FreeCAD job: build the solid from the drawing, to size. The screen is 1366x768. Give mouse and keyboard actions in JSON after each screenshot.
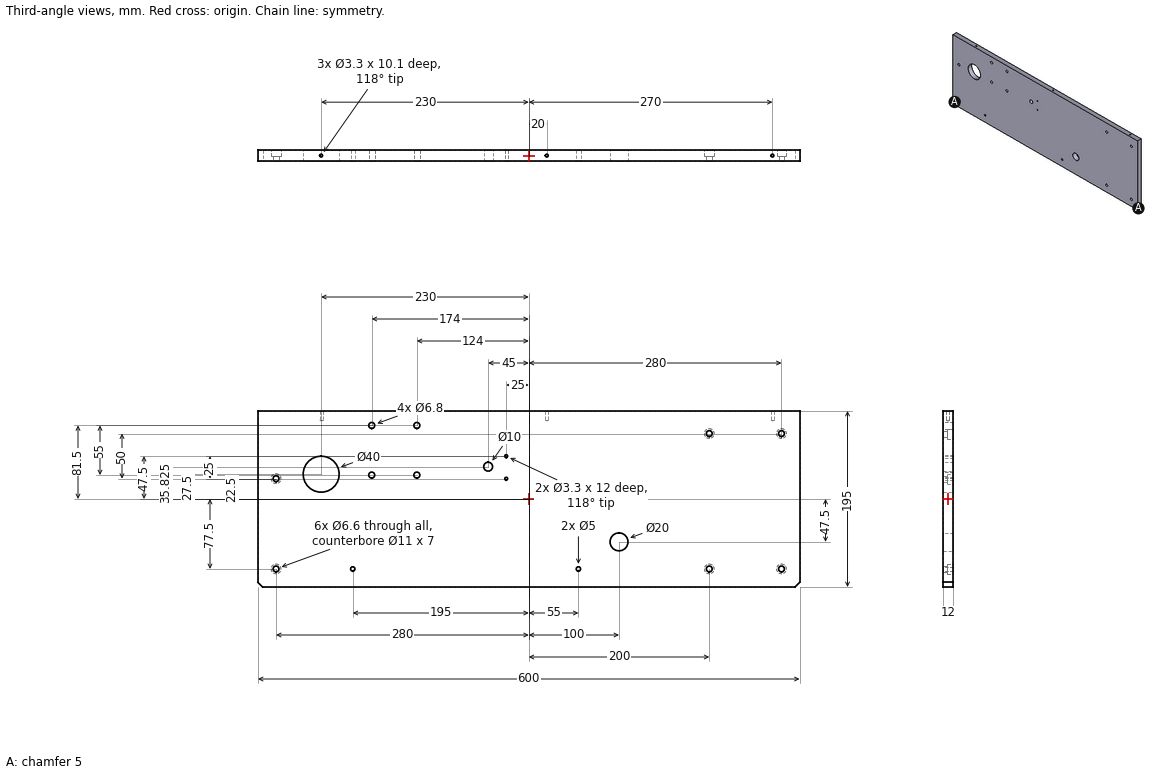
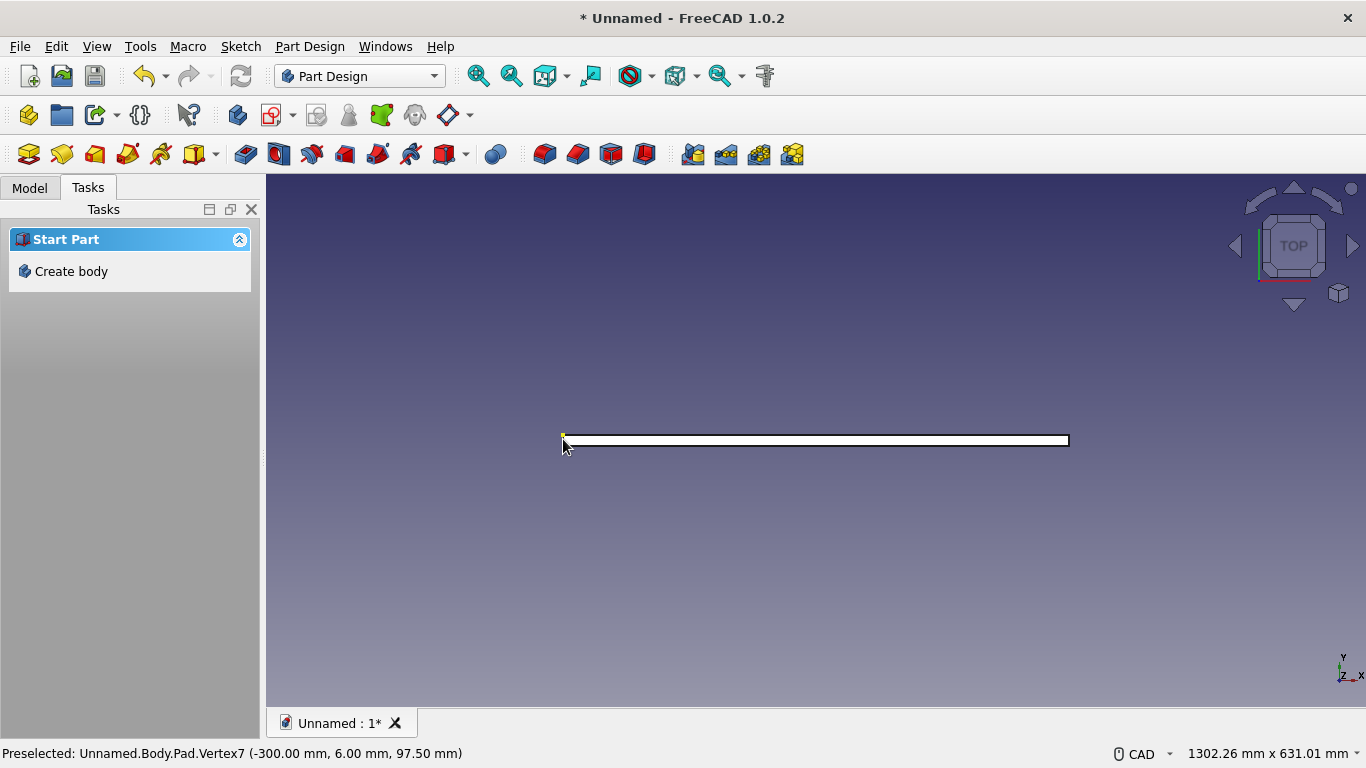
{"action": "key", "text": "1"}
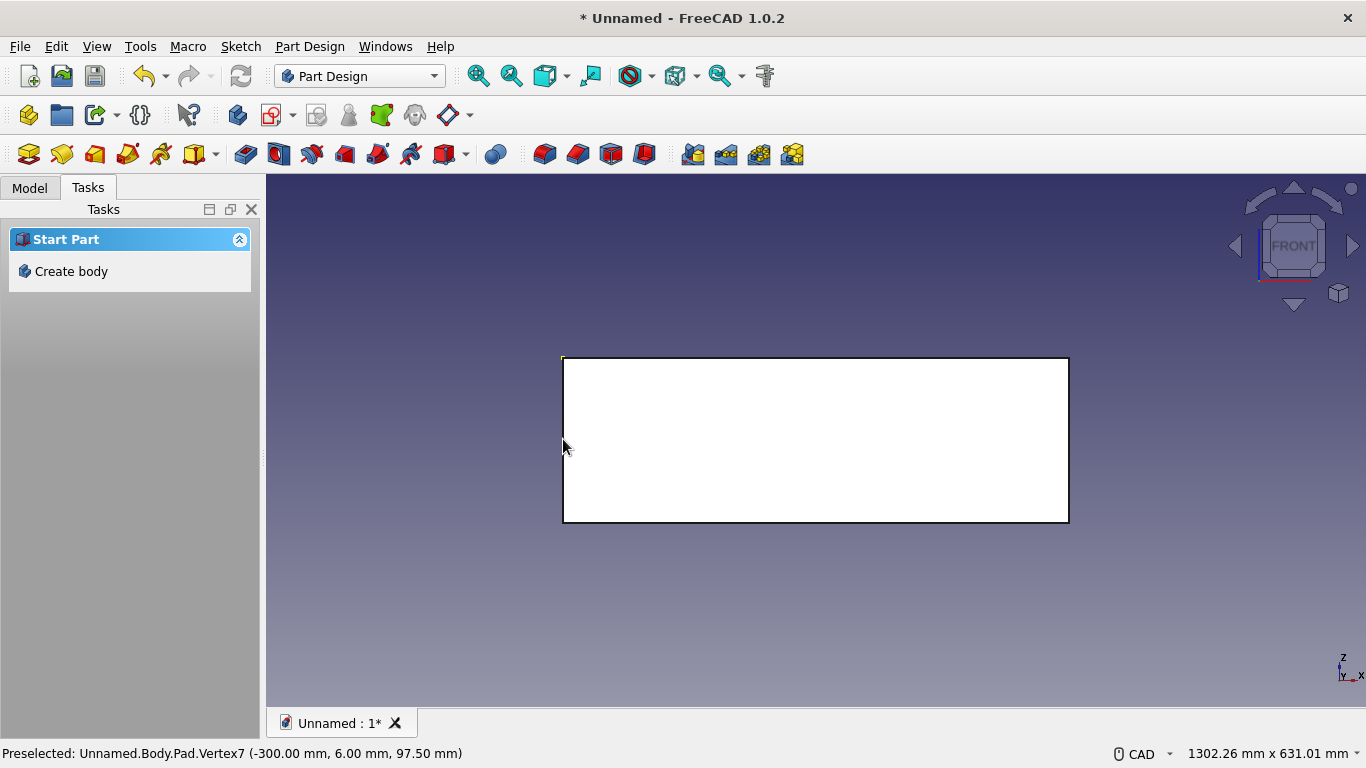
{"action": "scroll", "coordinate": [563, 522], "scroll_direction": "up", "scroll_amount": 7}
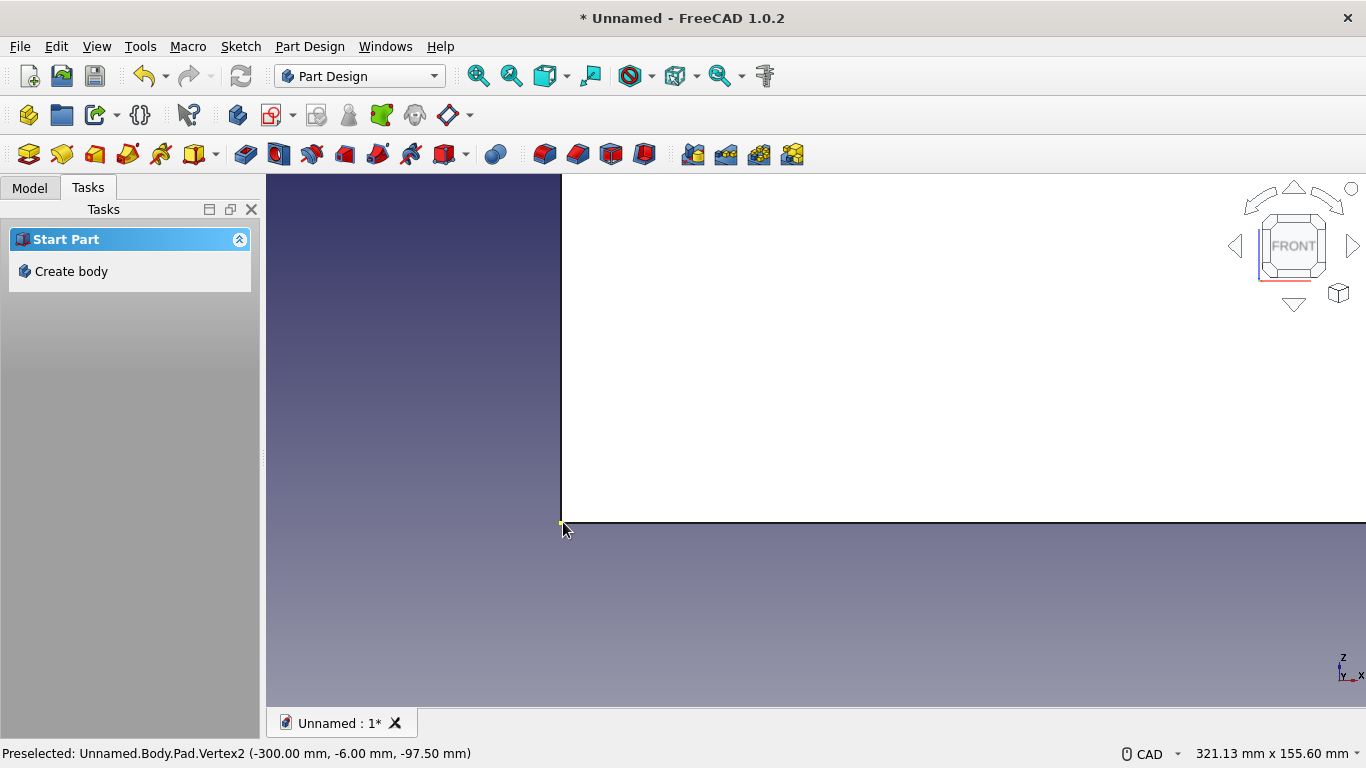
{"action": "key", "text": "v f"}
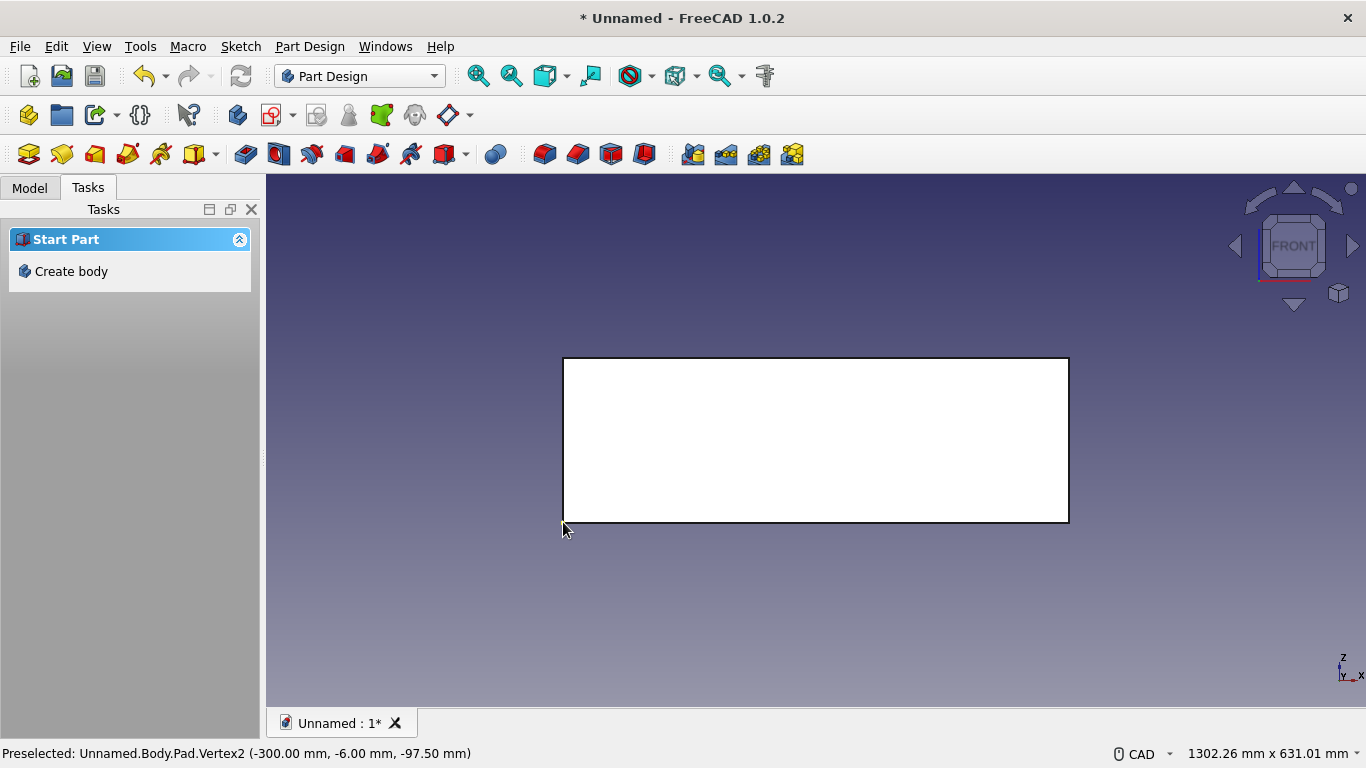
{"action": "key", "text": "3"}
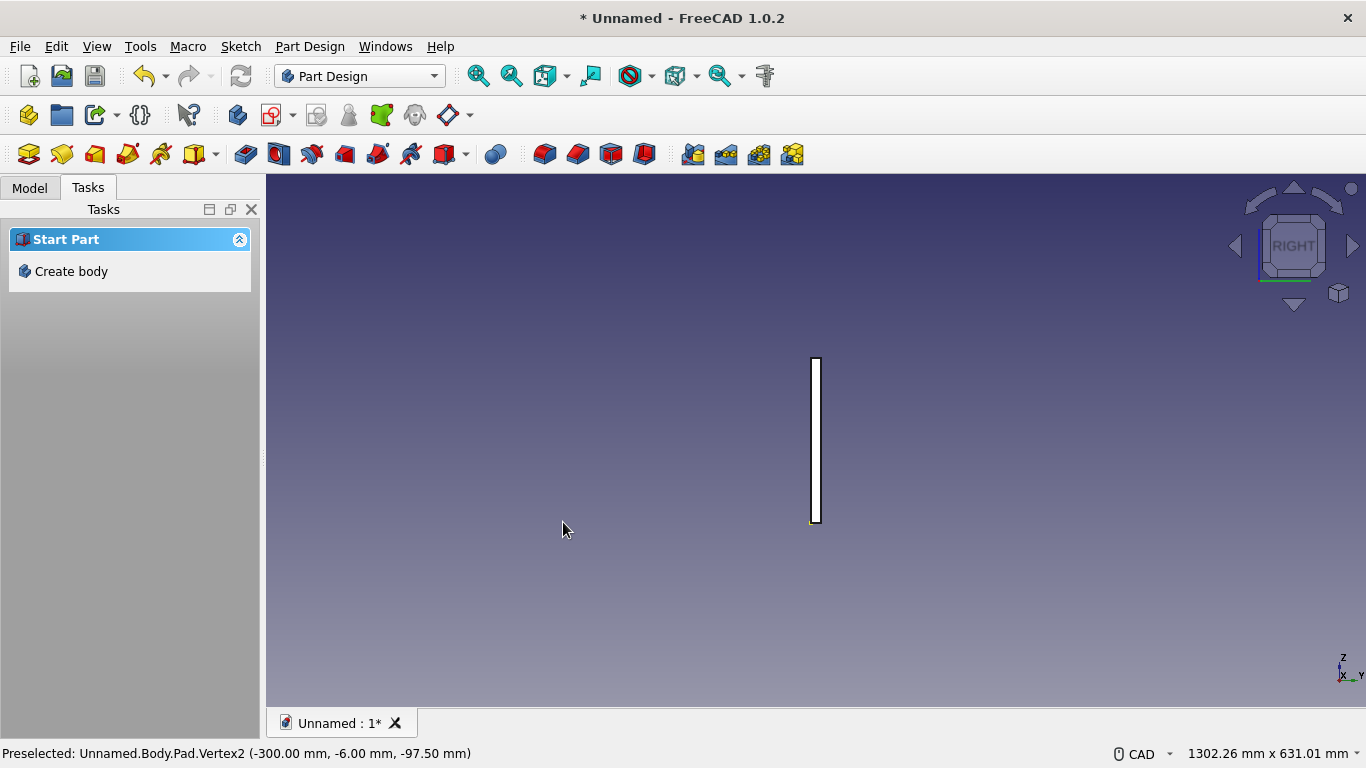
{"action": "key", "text": "v f"}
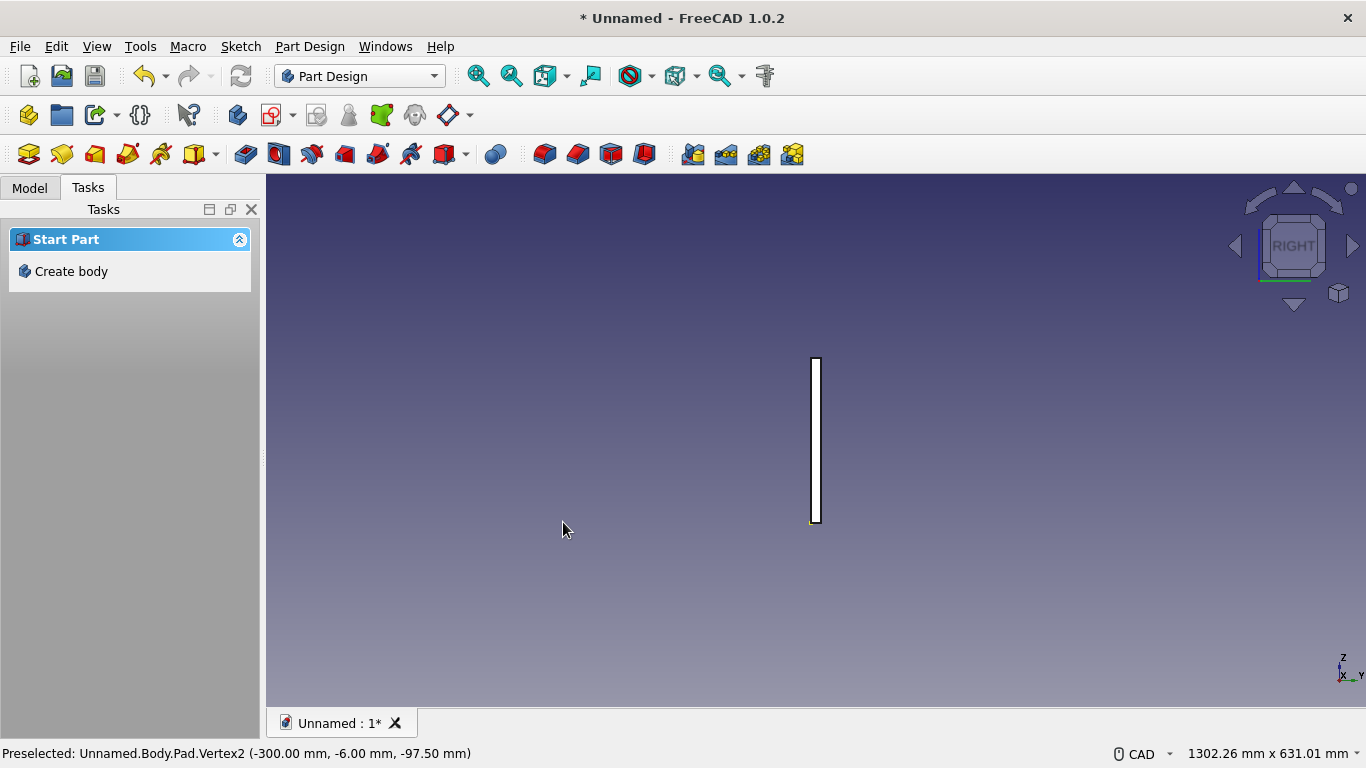
{"action": "scroll", "coordinate": [816, 522], "scroll_direction": "up", "scroll_amount": 7}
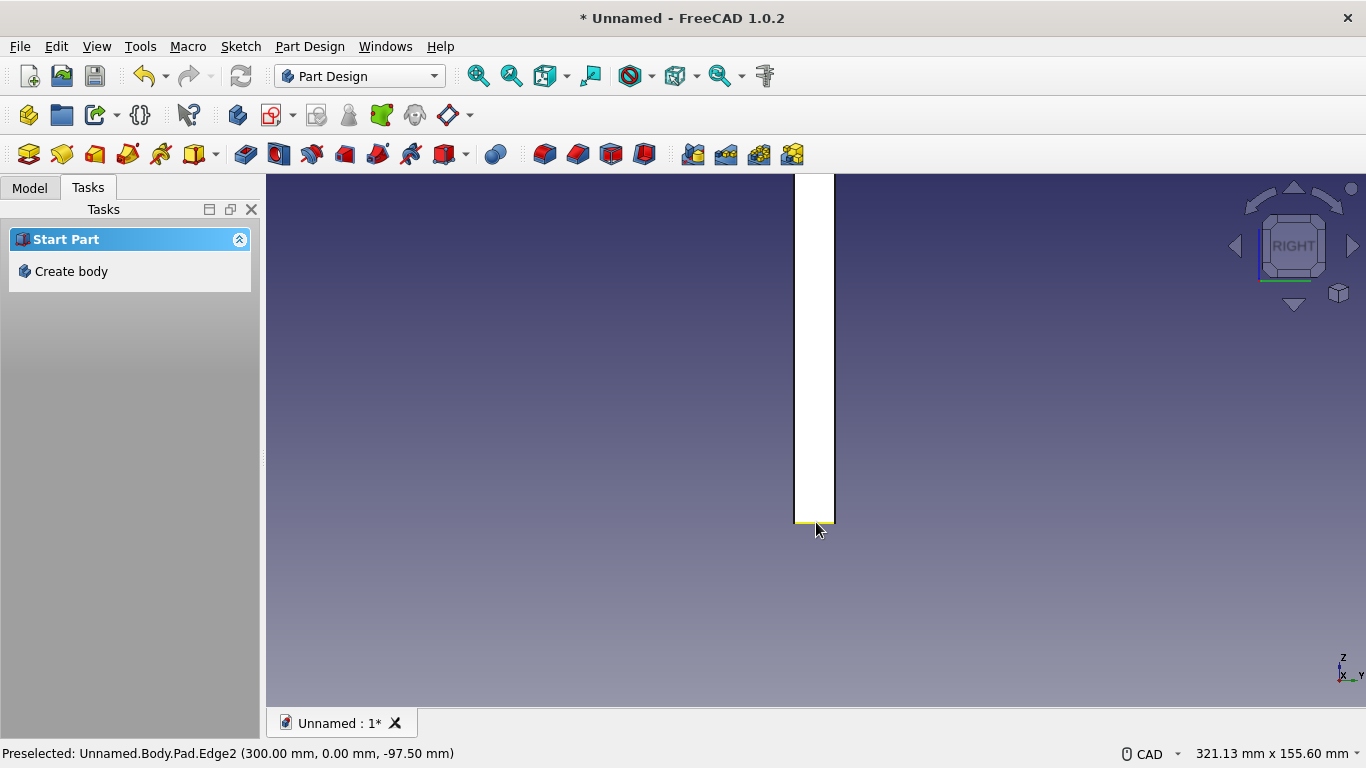
{"action": "left_click", "coordinate": [814, 522]}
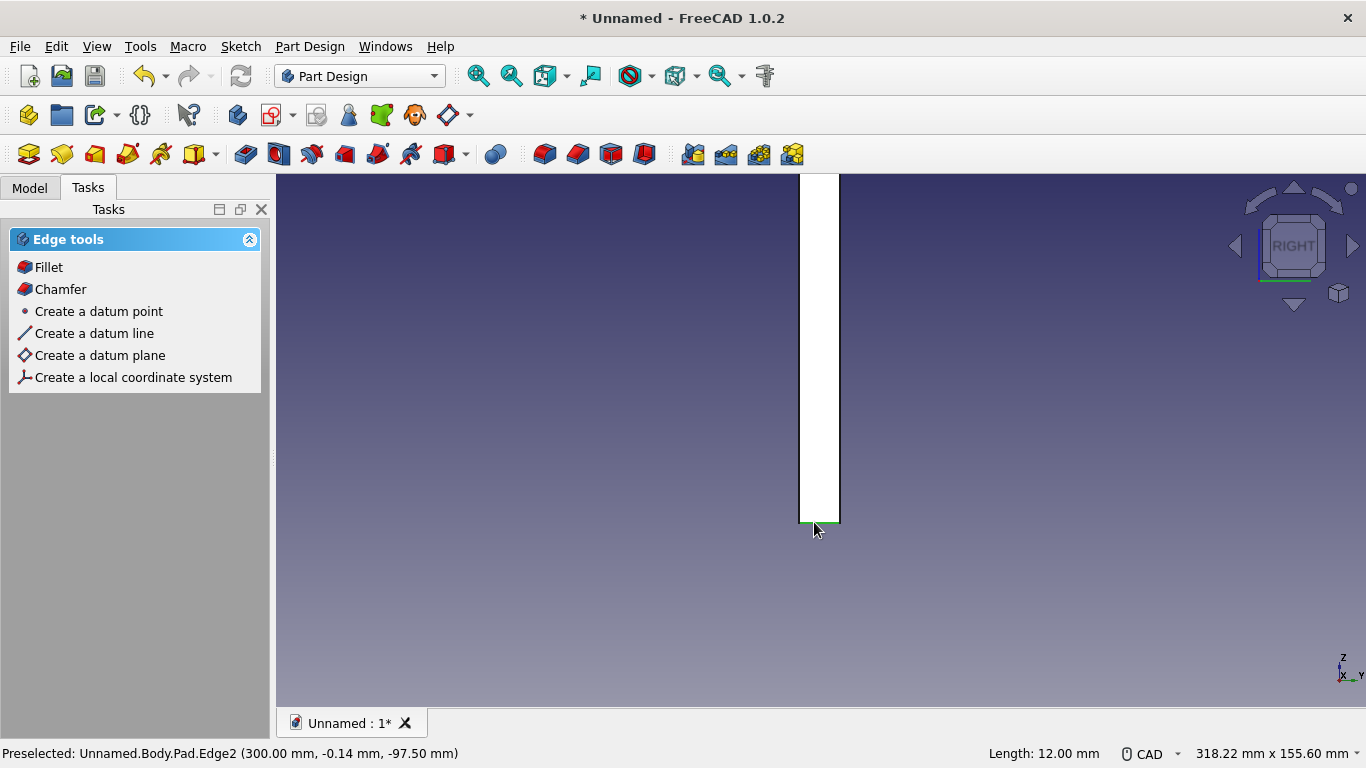
{"action": "key", "text": "v f"}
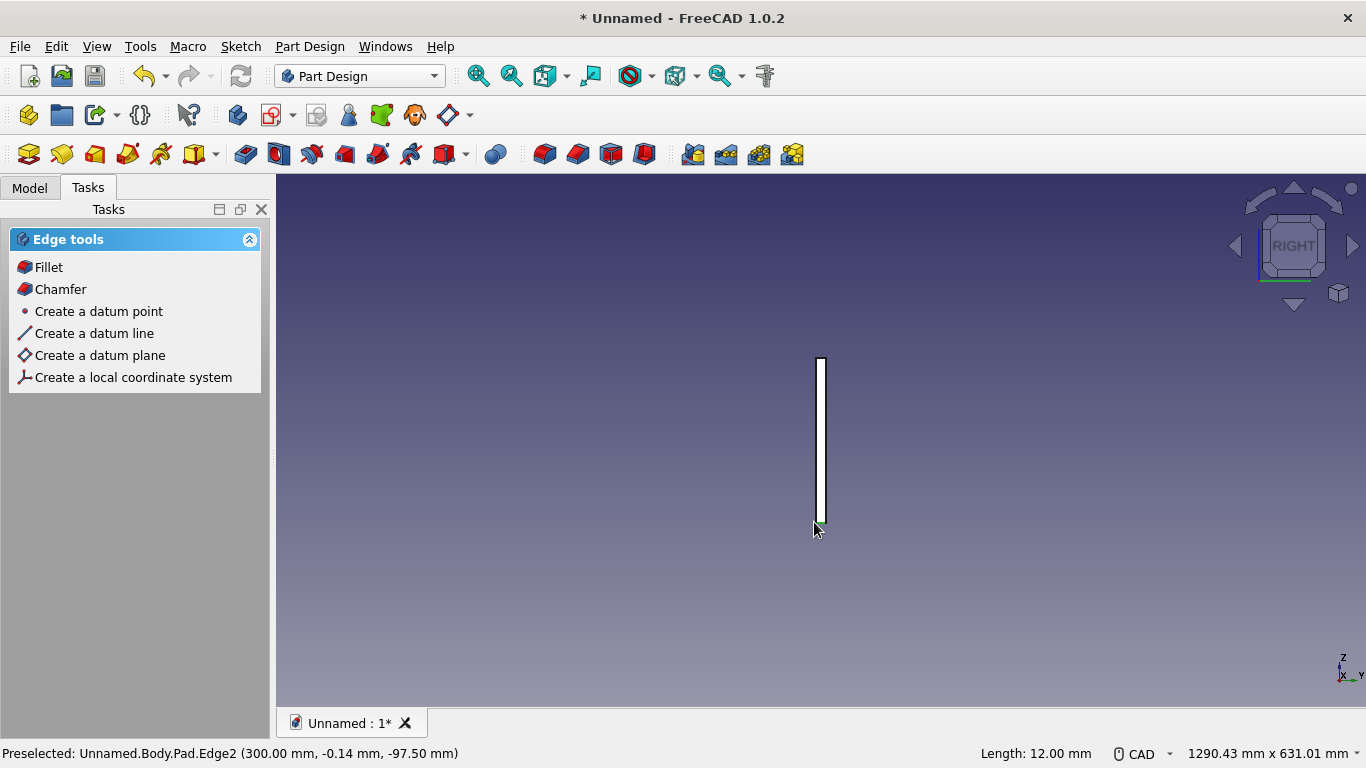
{"action": "key", "text": "5"}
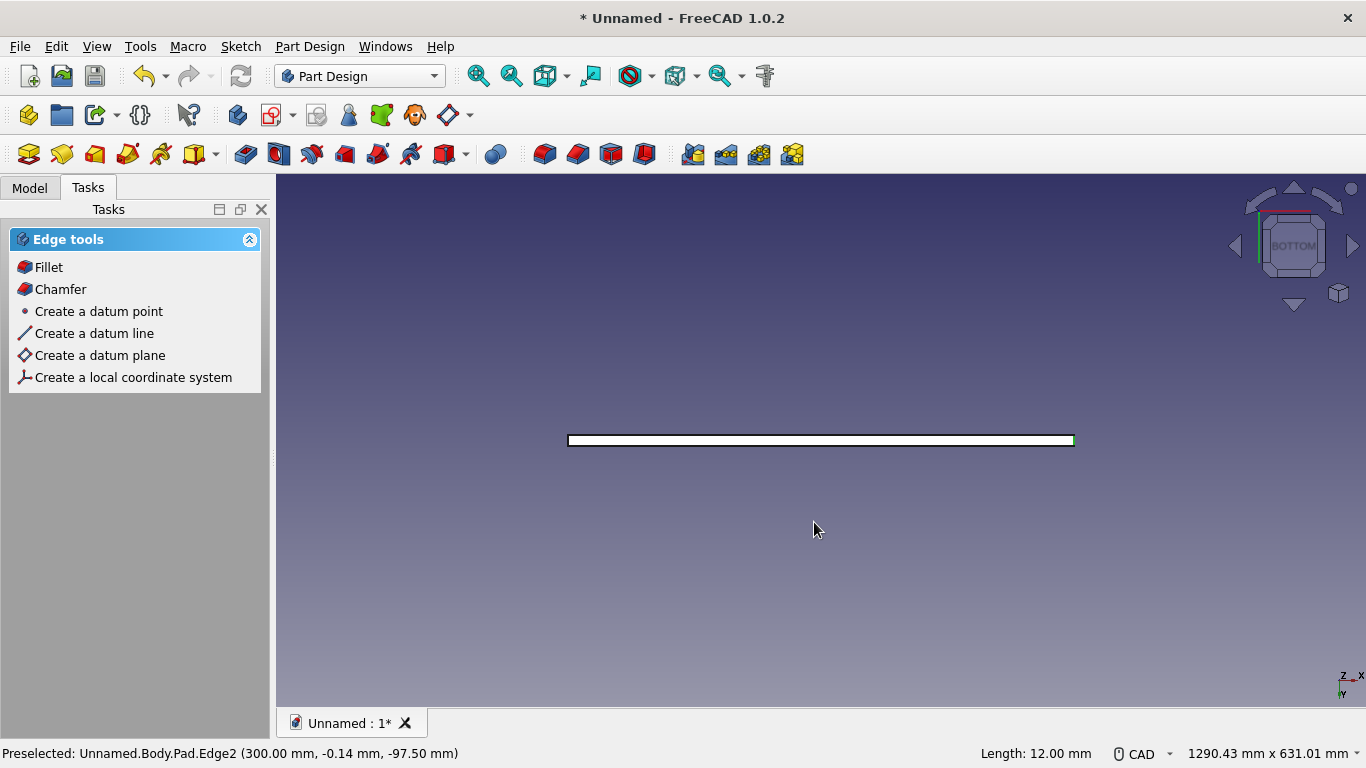
{"action": "left_click", "coordinate": [568, 441], "text": "ctrl"}